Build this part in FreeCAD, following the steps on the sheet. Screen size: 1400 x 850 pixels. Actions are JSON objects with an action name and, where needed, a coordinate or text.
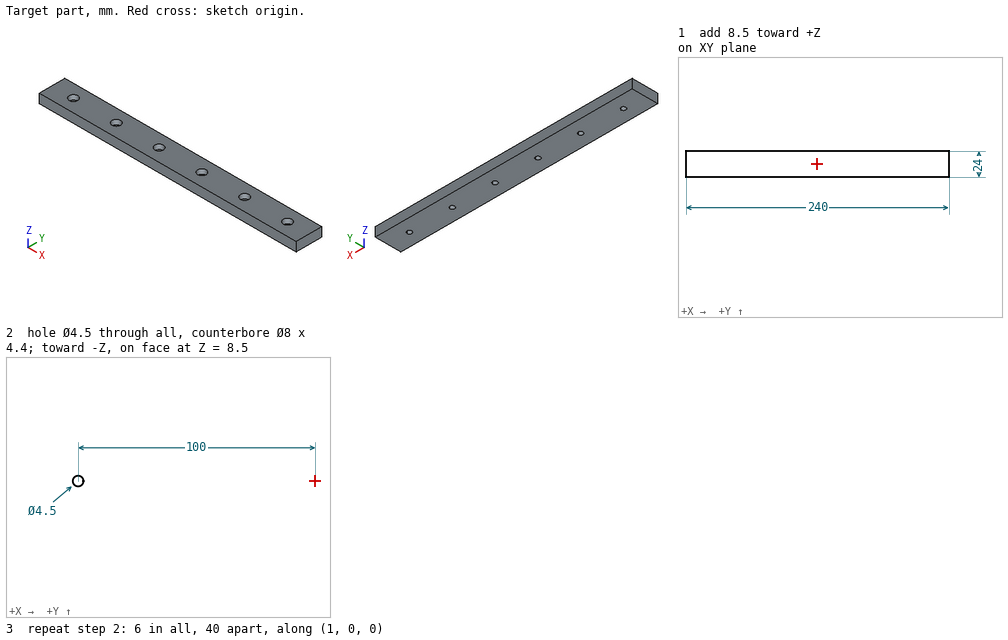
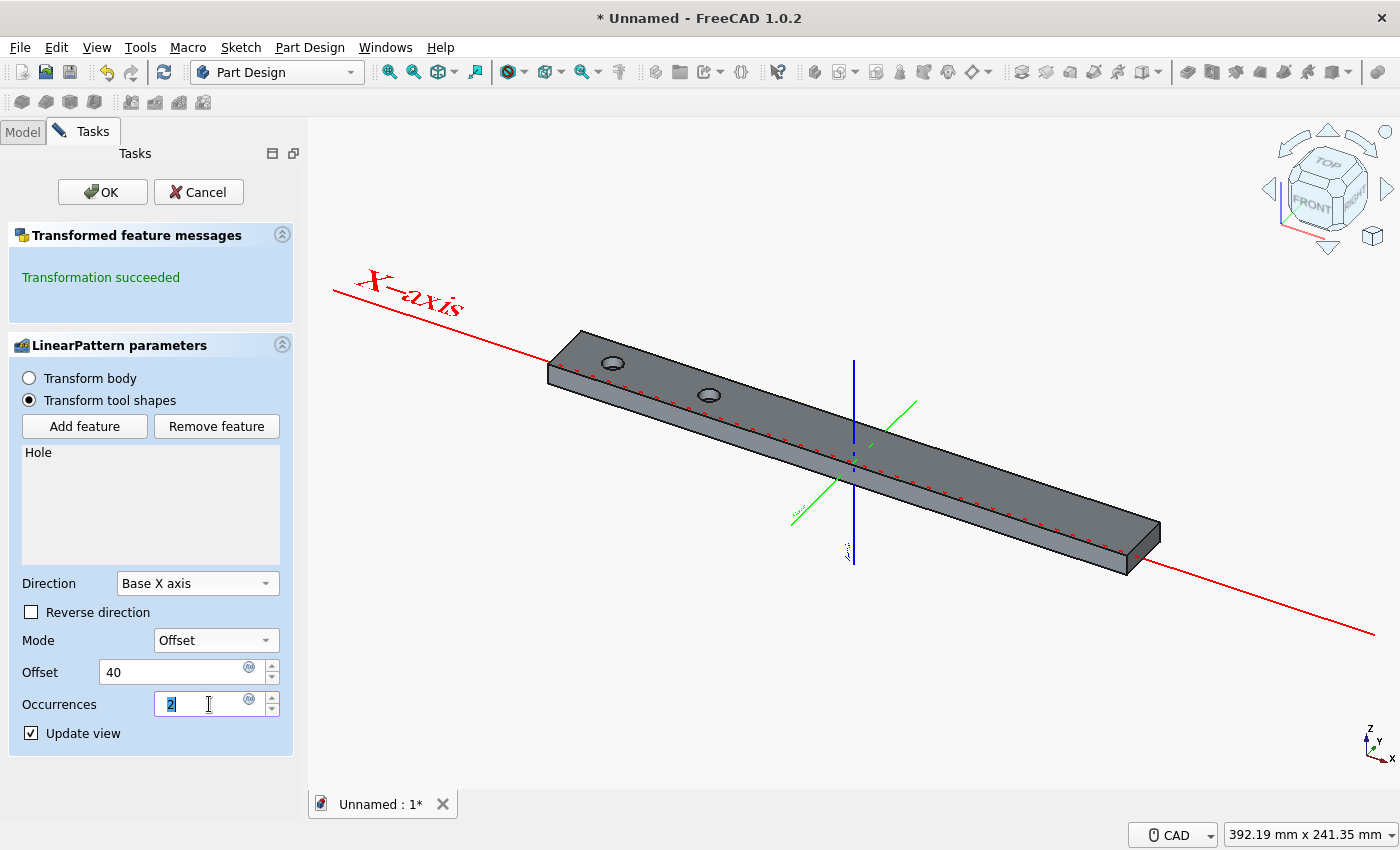
{"action": "type", "text": "6"}
{"action": "key", "text": "Tab"}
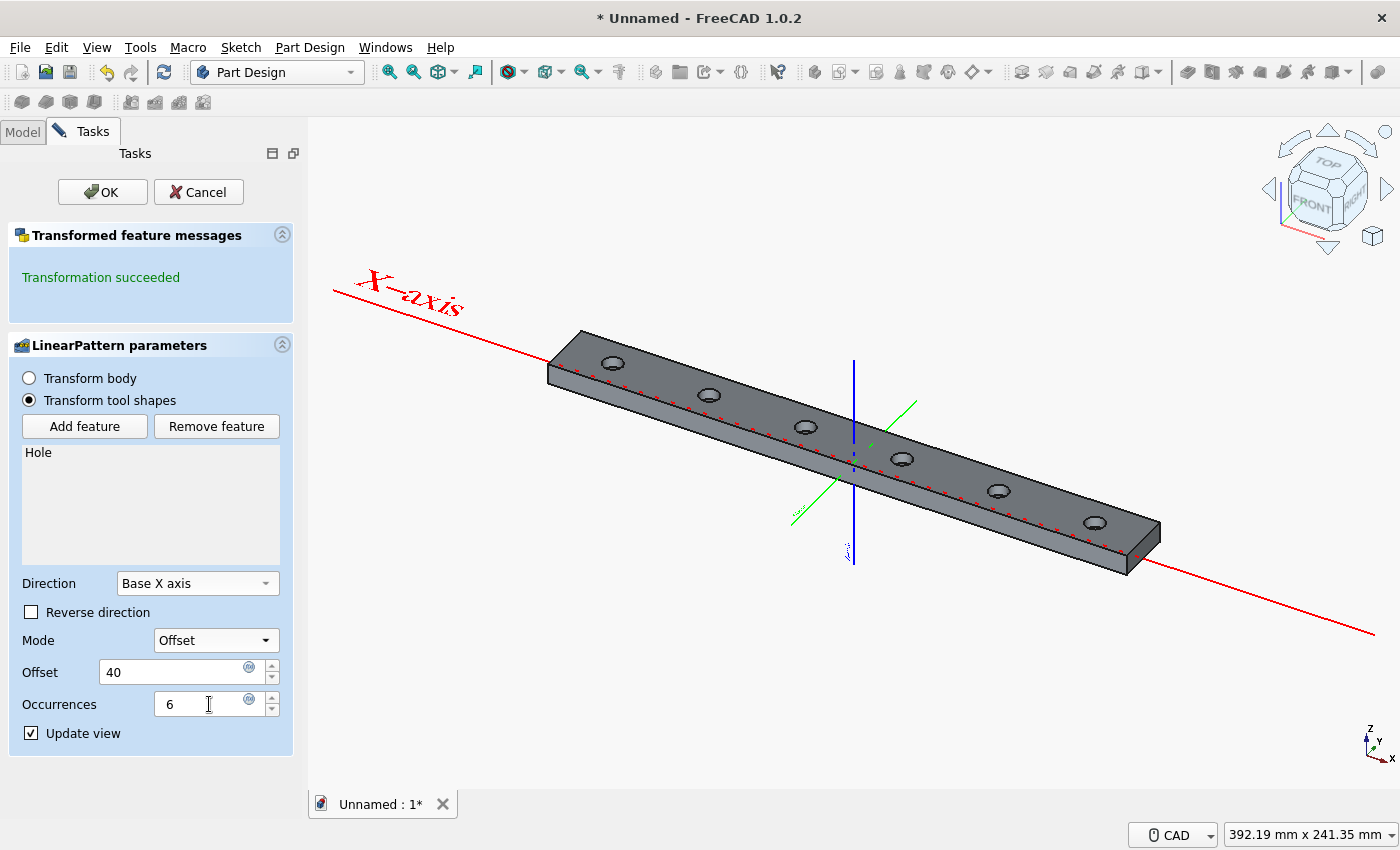
{"action": "left_click", "coordinate": [103, 192]}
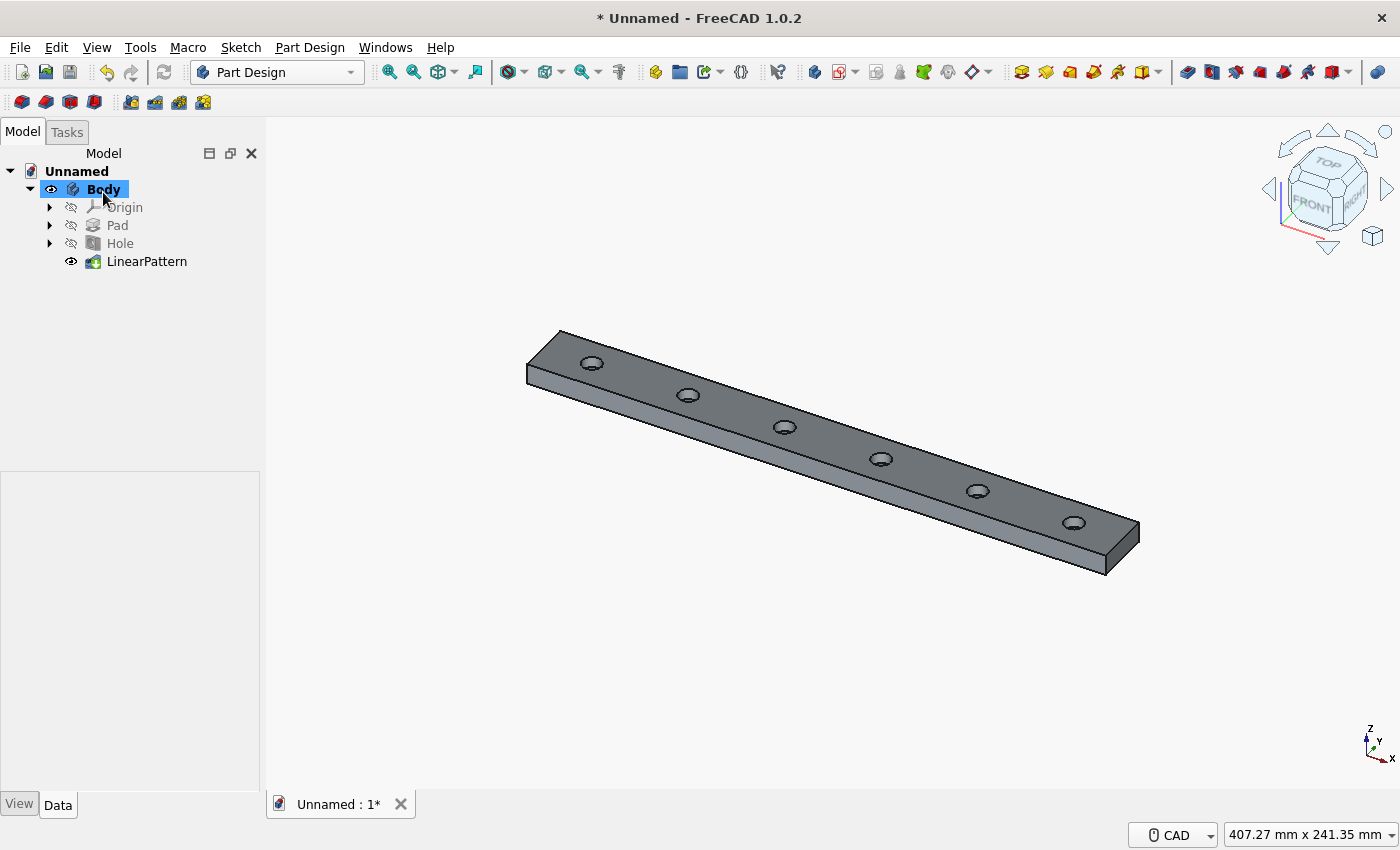
{"action": "key", "text": "0"}